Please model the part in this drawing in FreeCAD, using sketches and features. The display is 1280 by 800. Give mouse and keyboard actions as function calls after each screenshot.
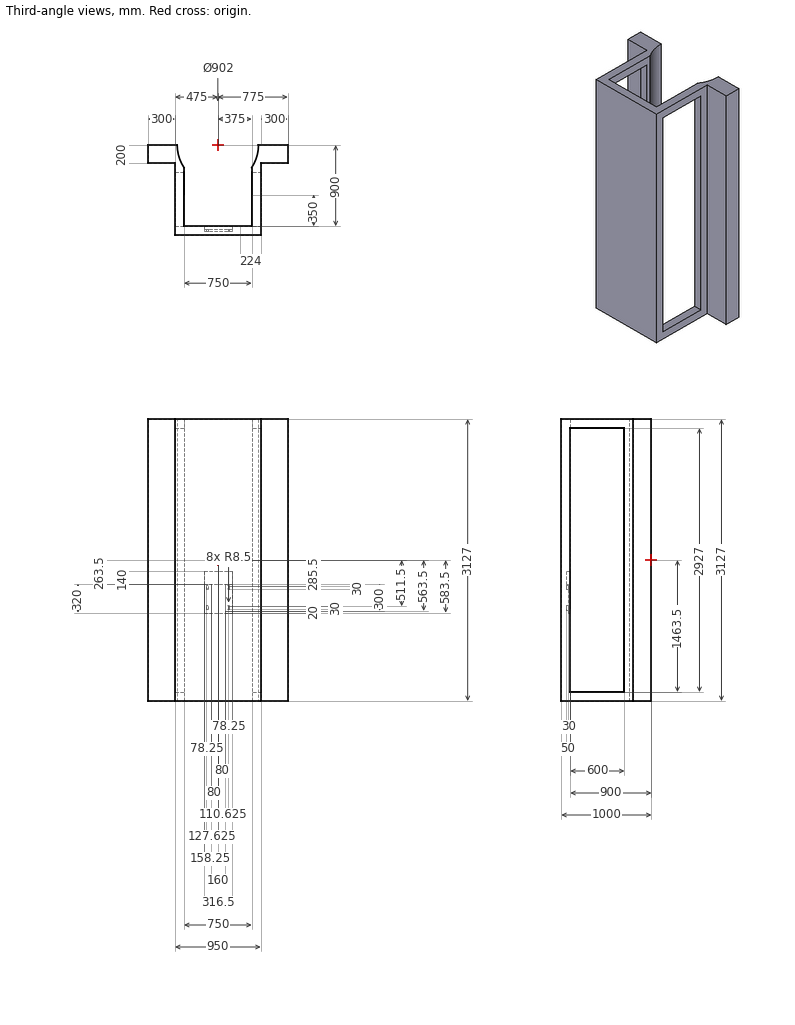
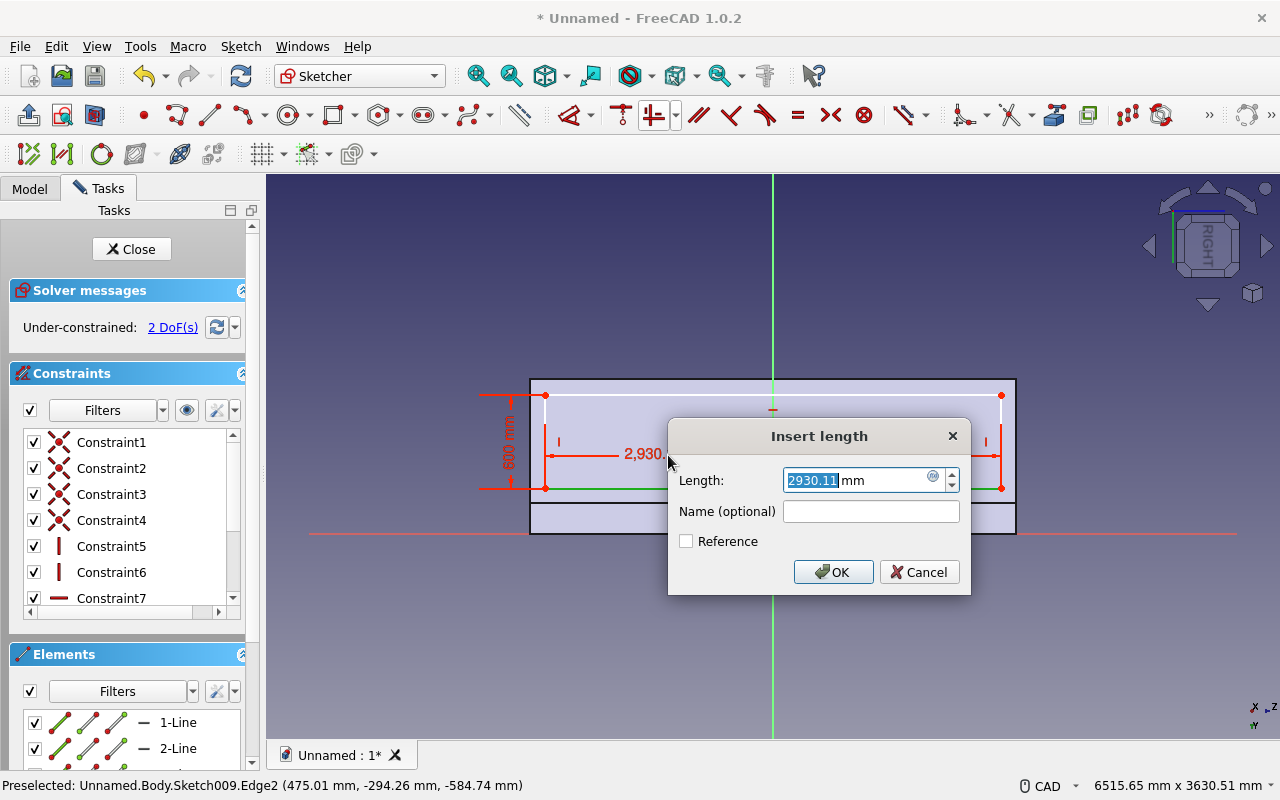
text(2927)
key(Return)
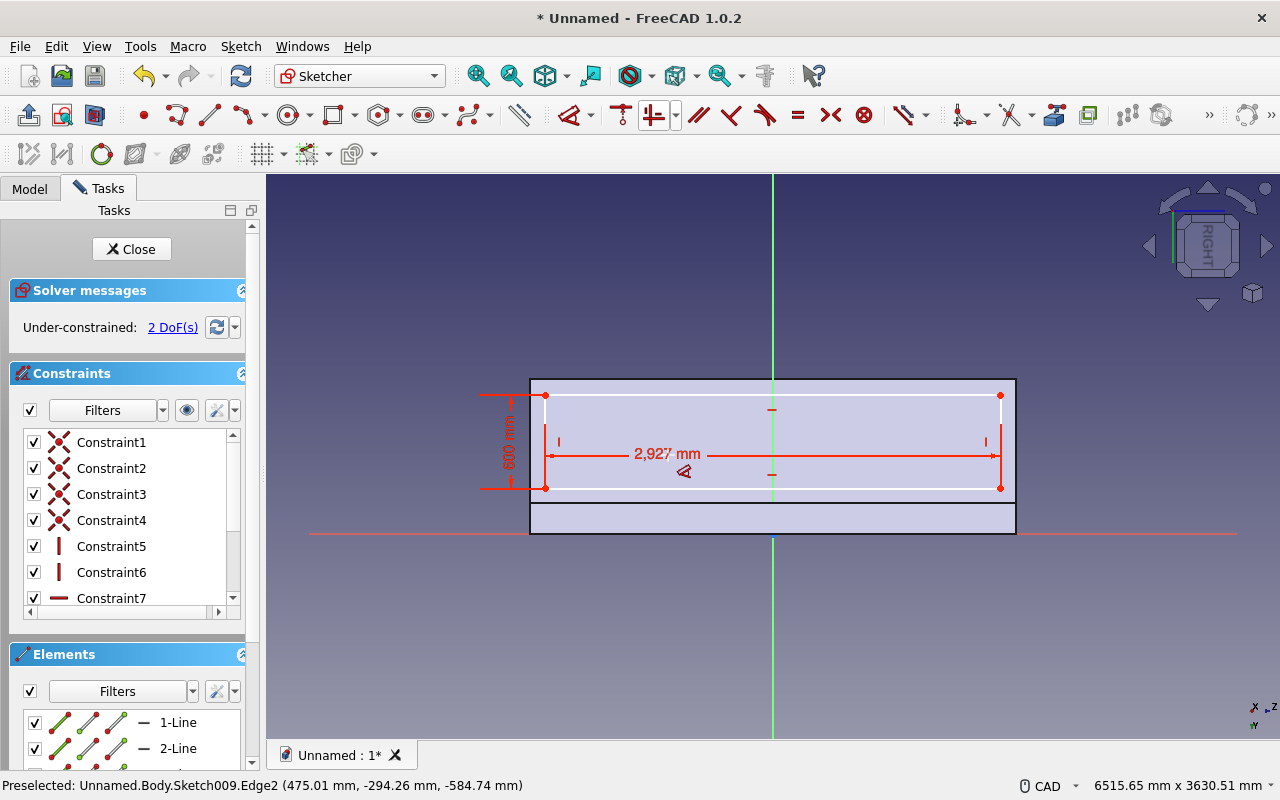
click(545, 395)
click(511, 465)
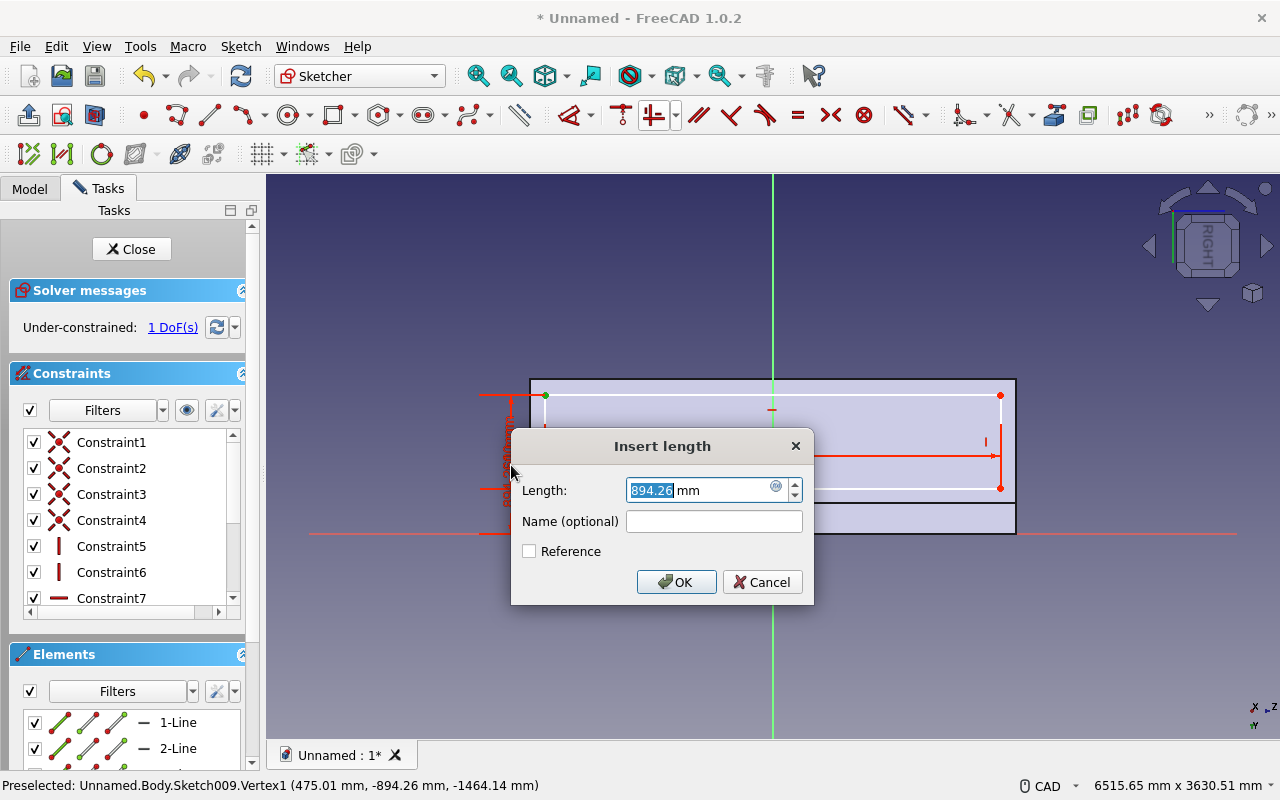
text(900)
key(Return)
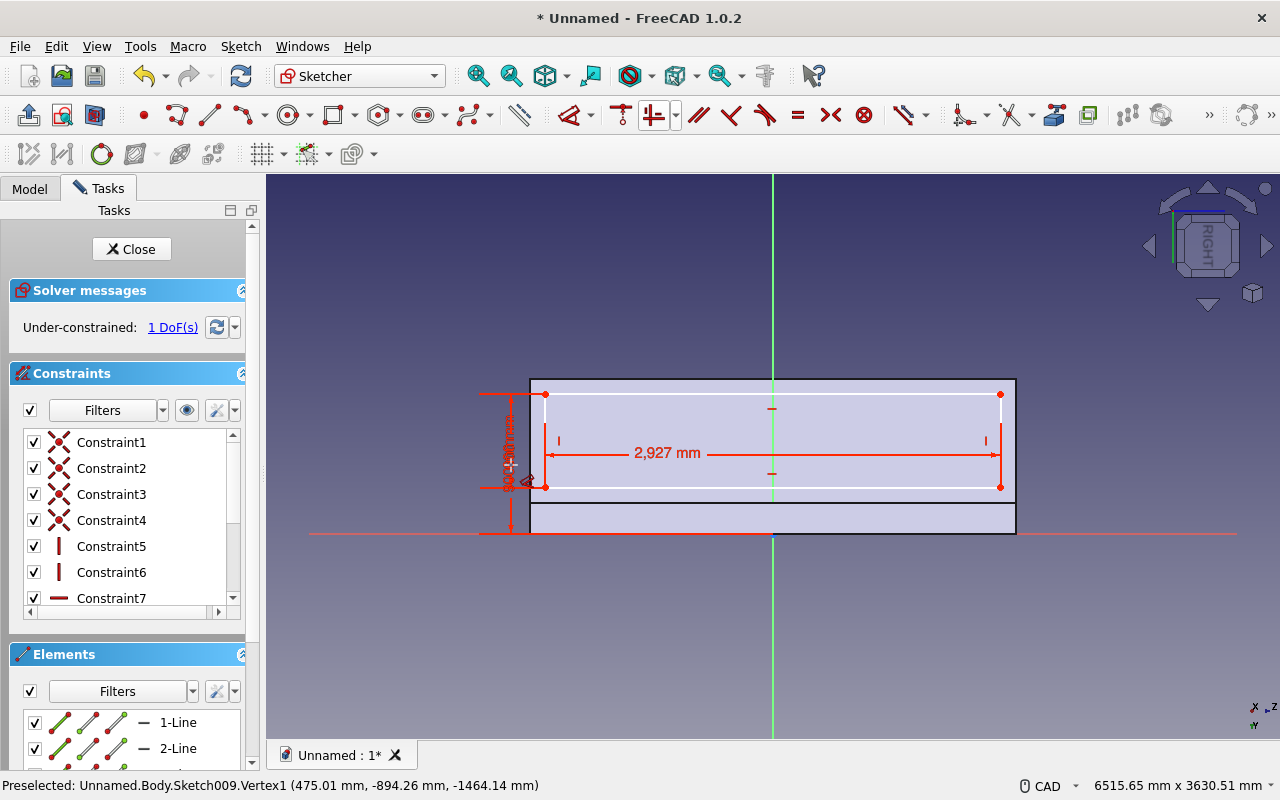
click(545, 394)
click(659, 568)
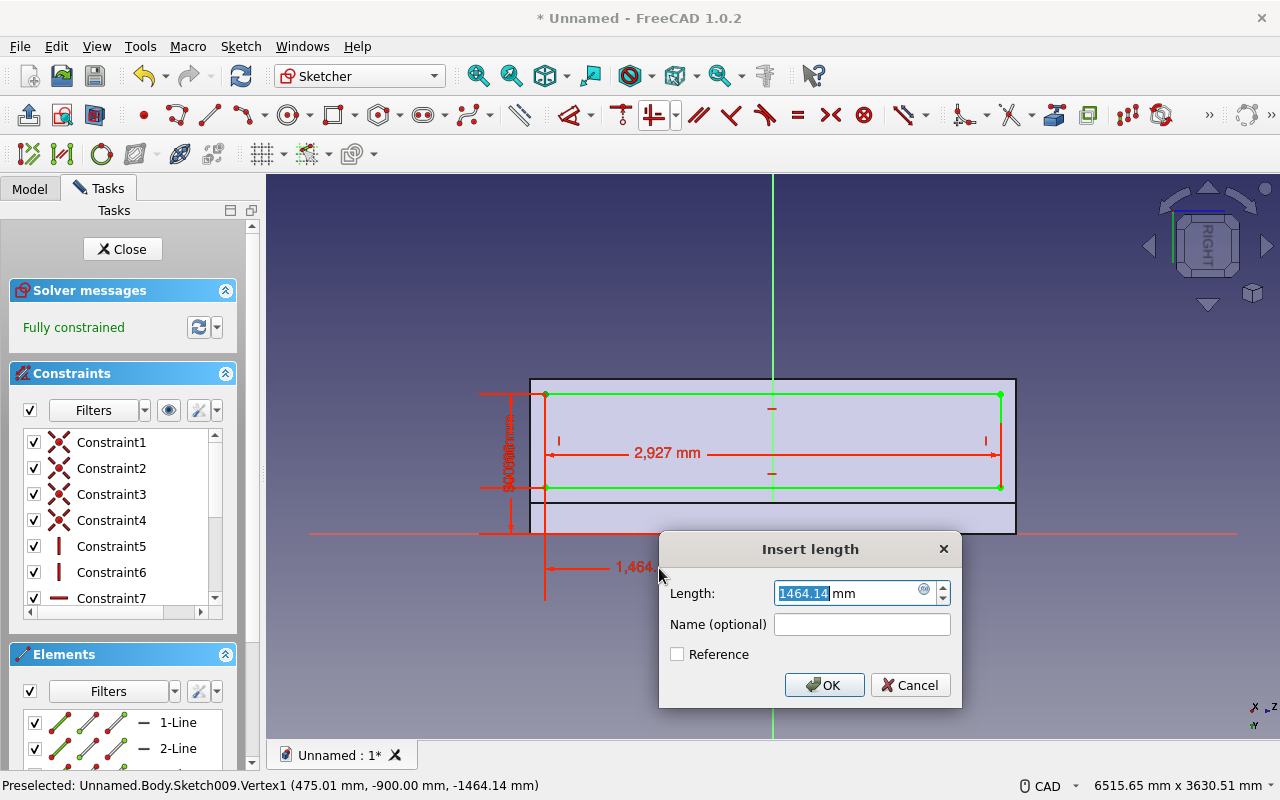
text(1463.5)
key(Return)
key(Escape)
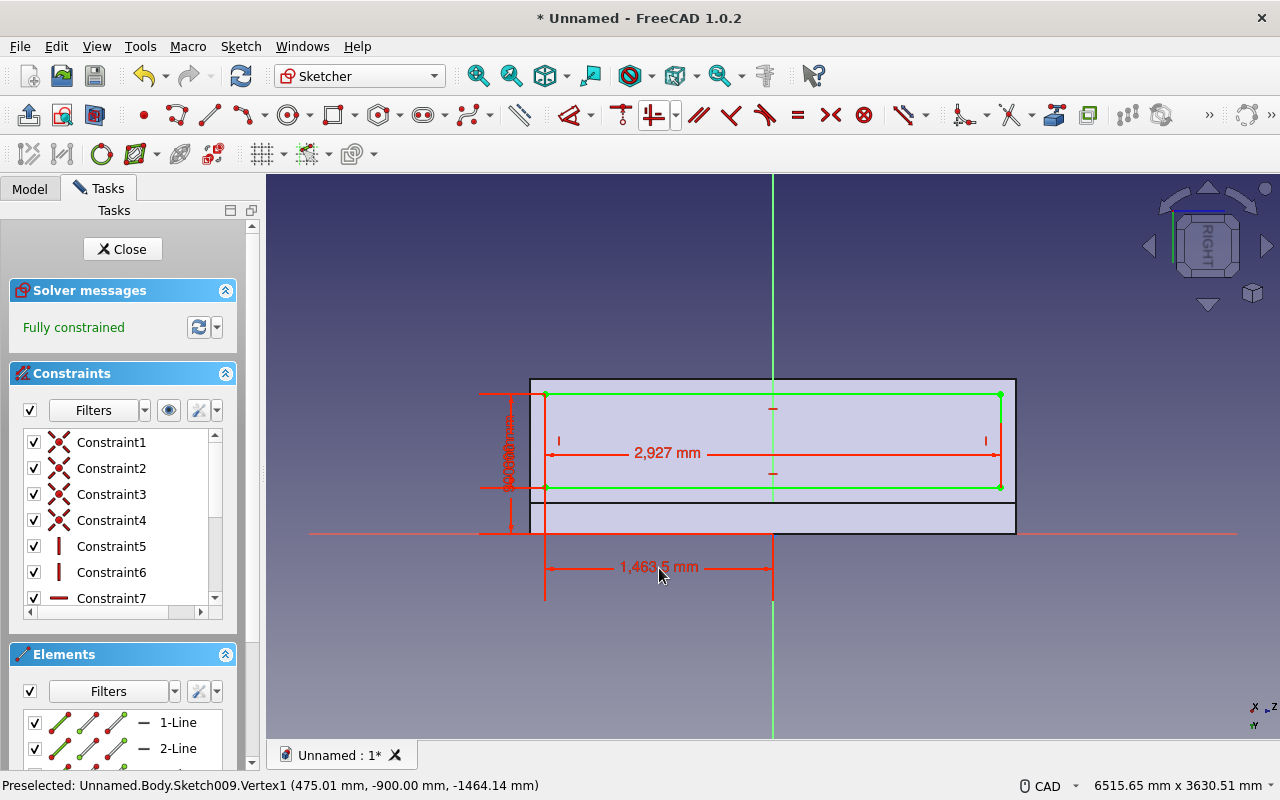
click(123, 249)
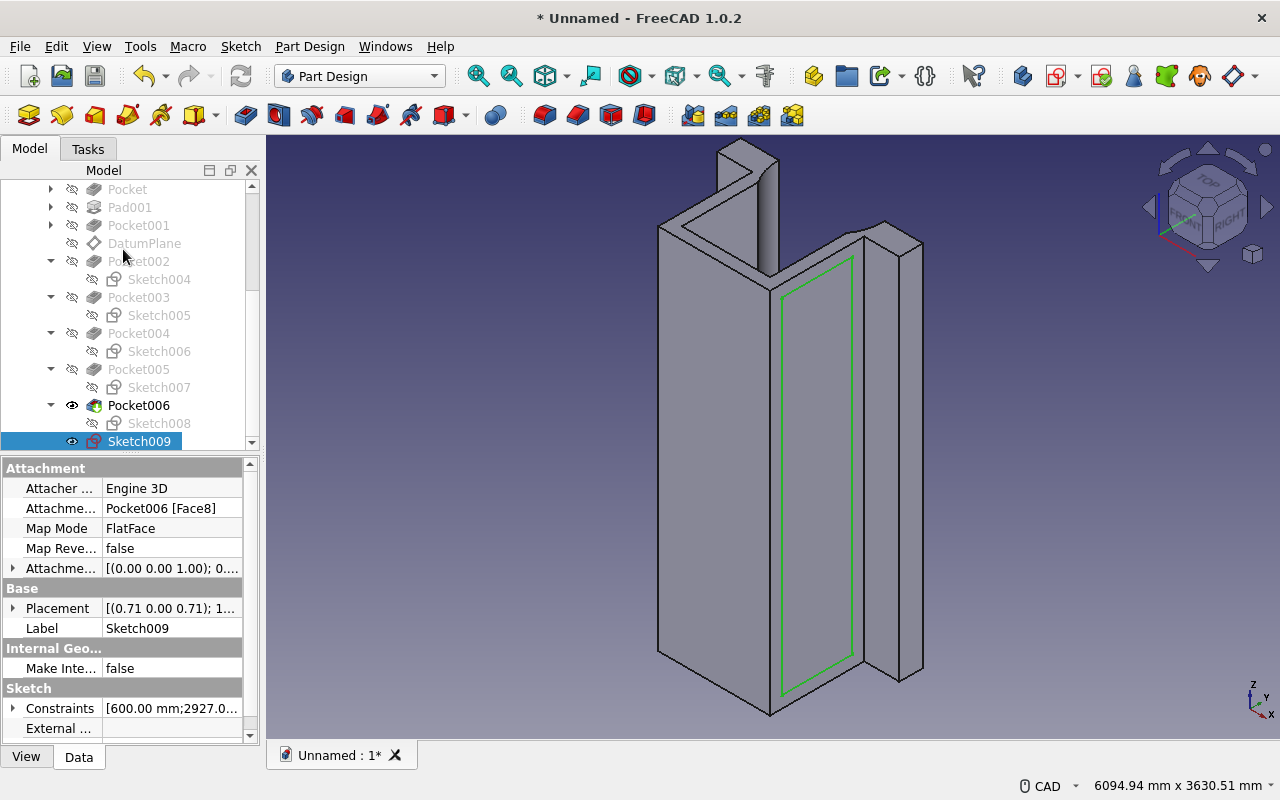
click(246, 116)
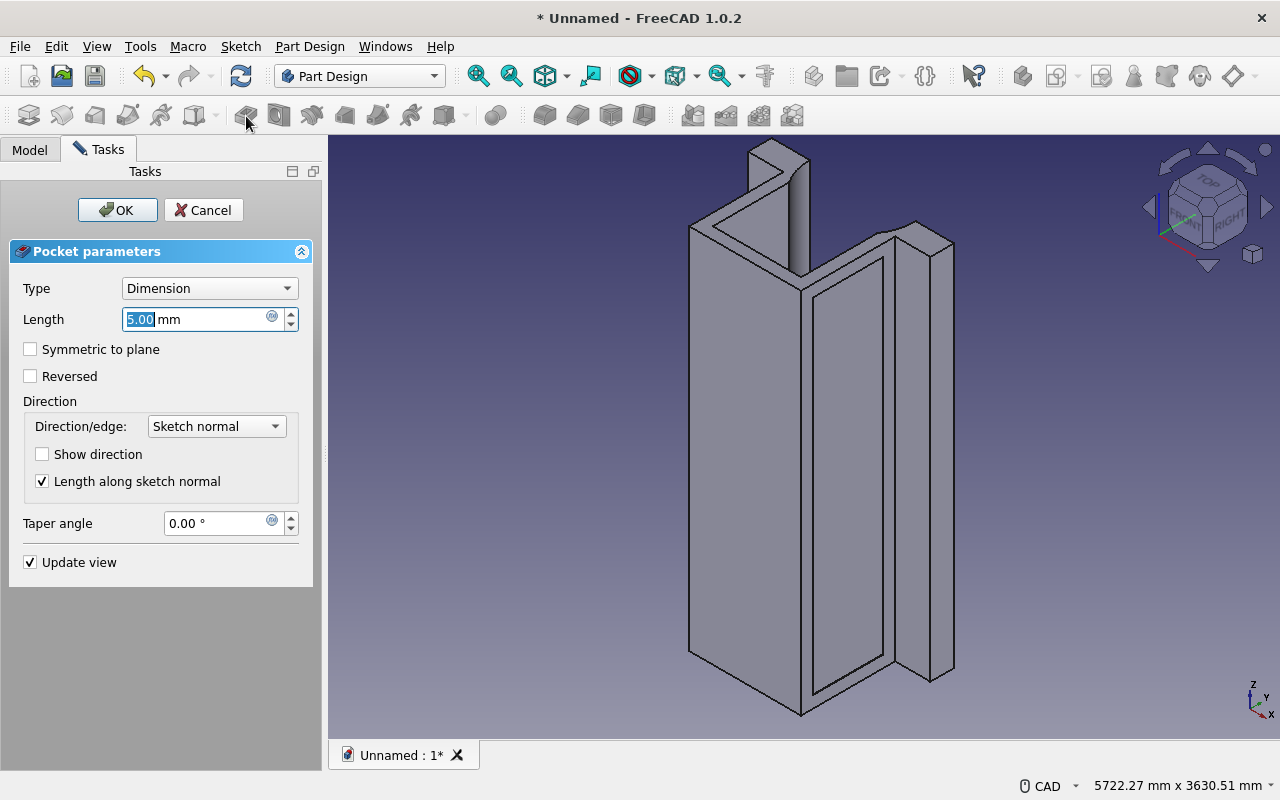
text(224)
key(Tab)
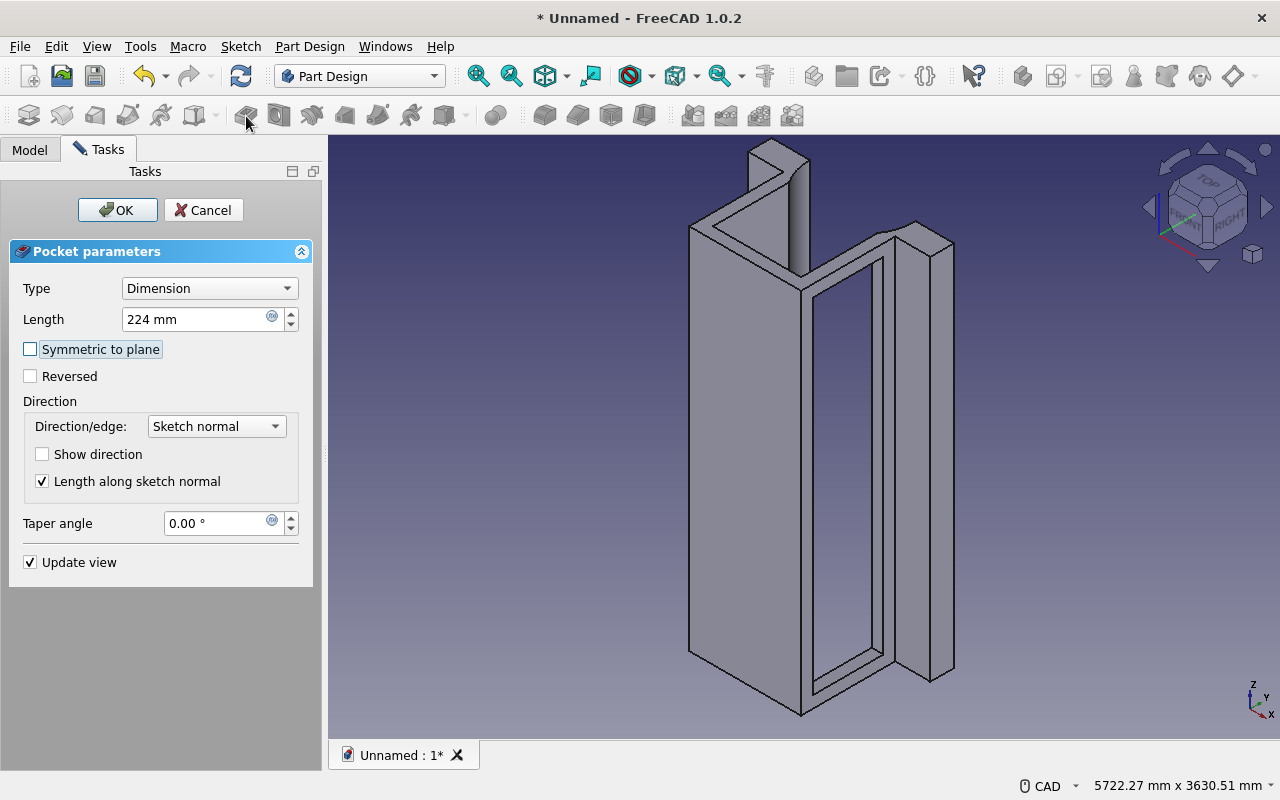
click(118, 210)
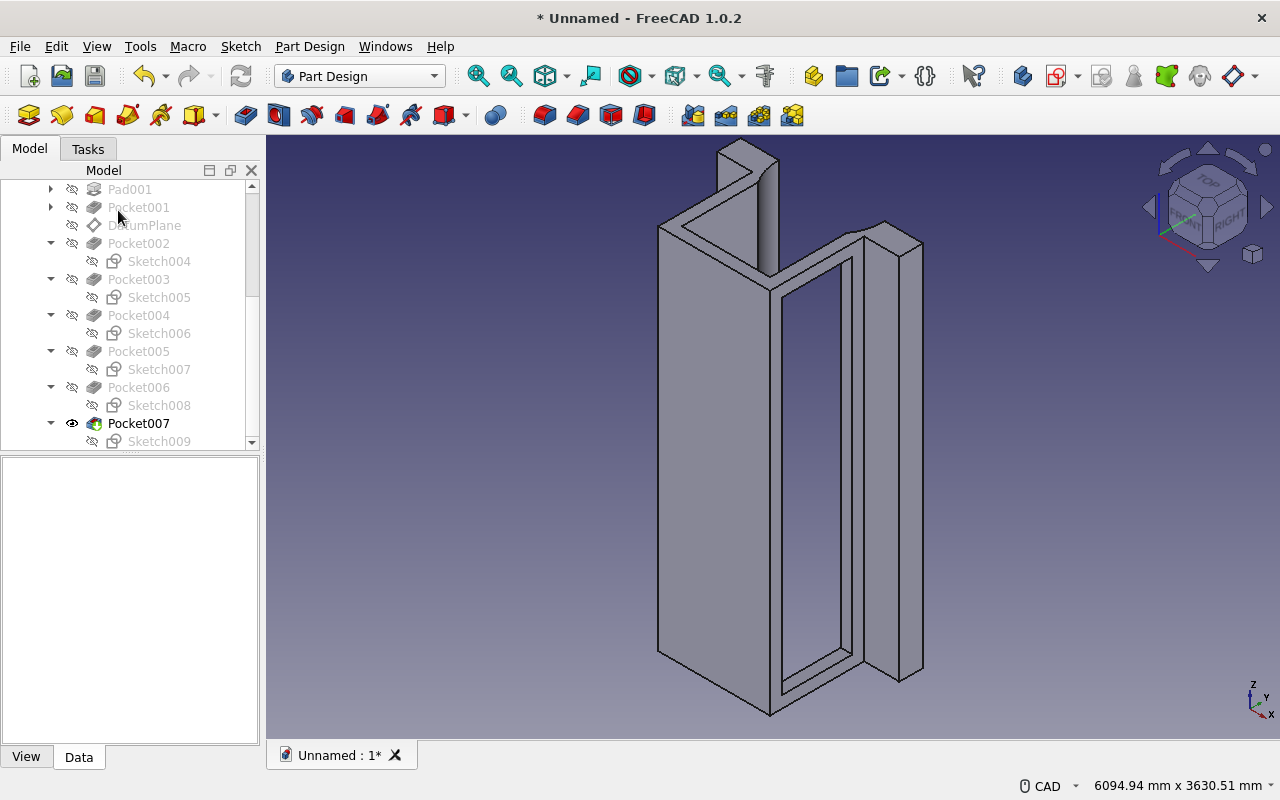
click(117, 423)